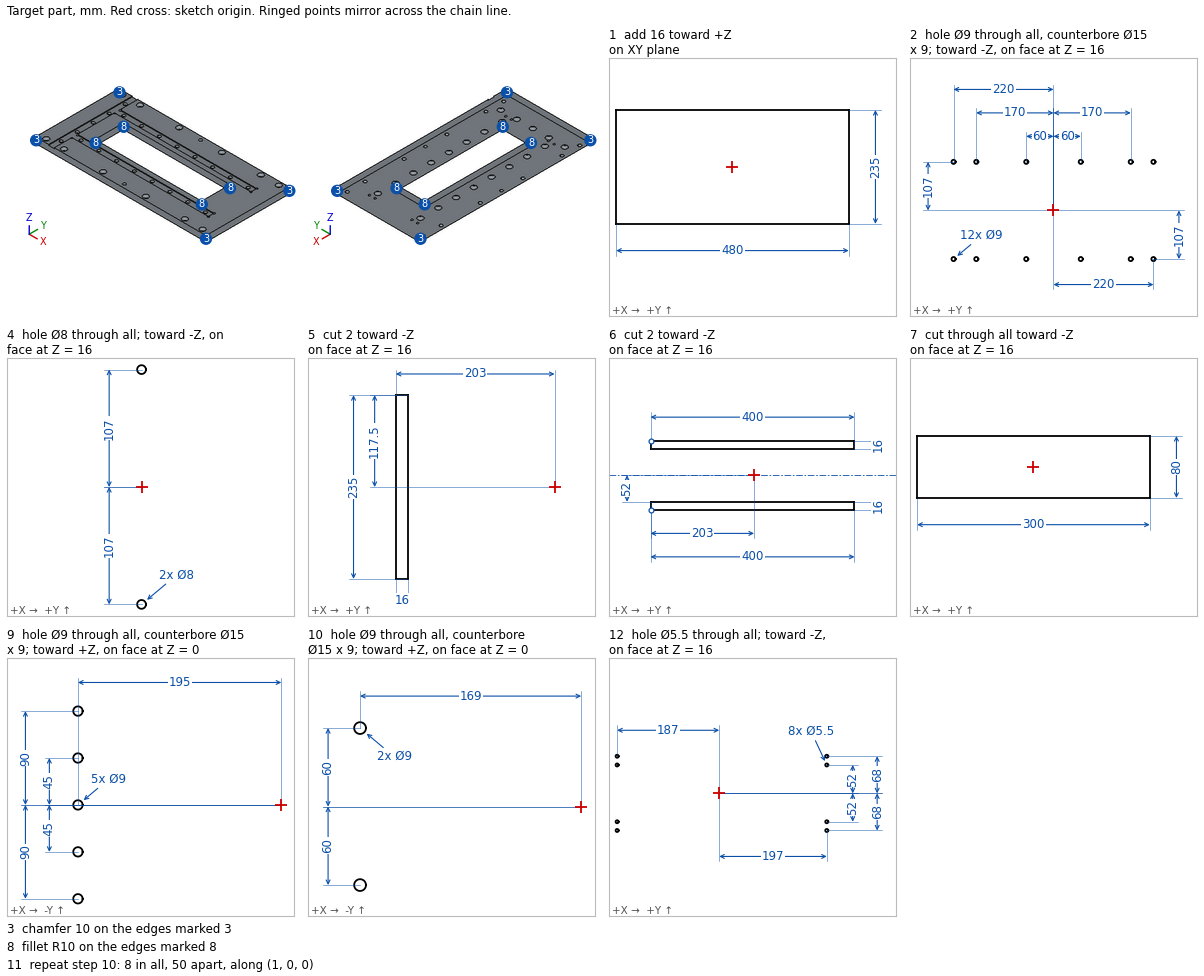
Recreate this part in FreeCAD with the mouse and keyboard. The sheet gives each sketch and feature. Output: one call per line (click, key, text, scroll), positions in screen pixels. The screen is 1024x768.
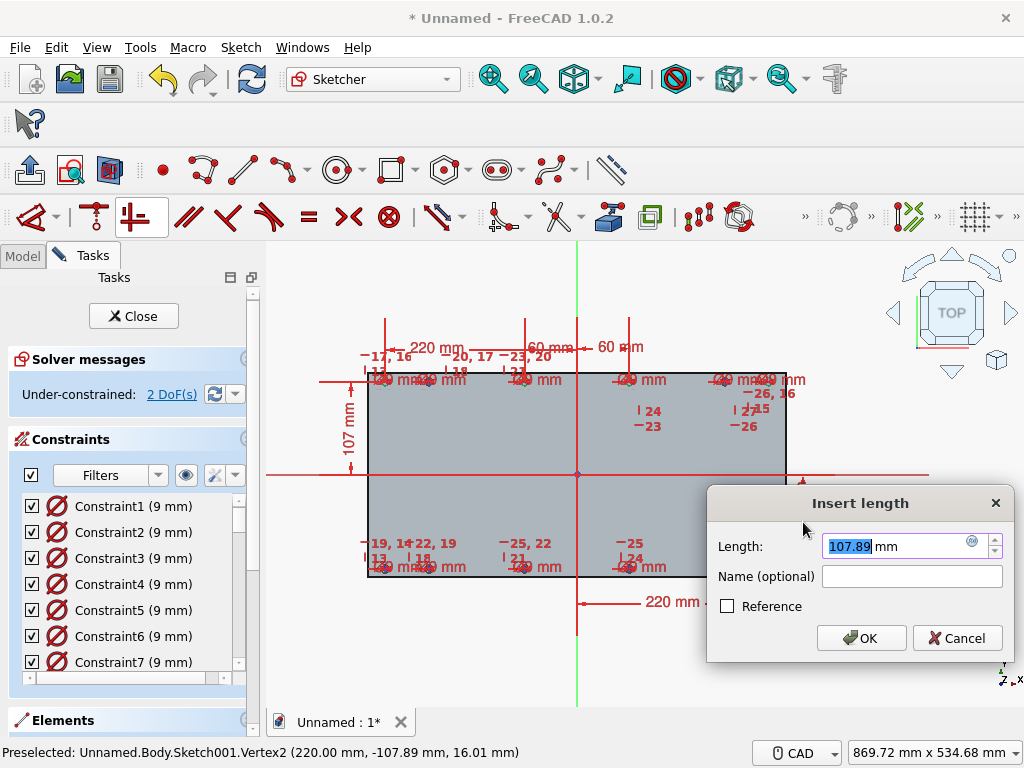
text(107)
key(Return)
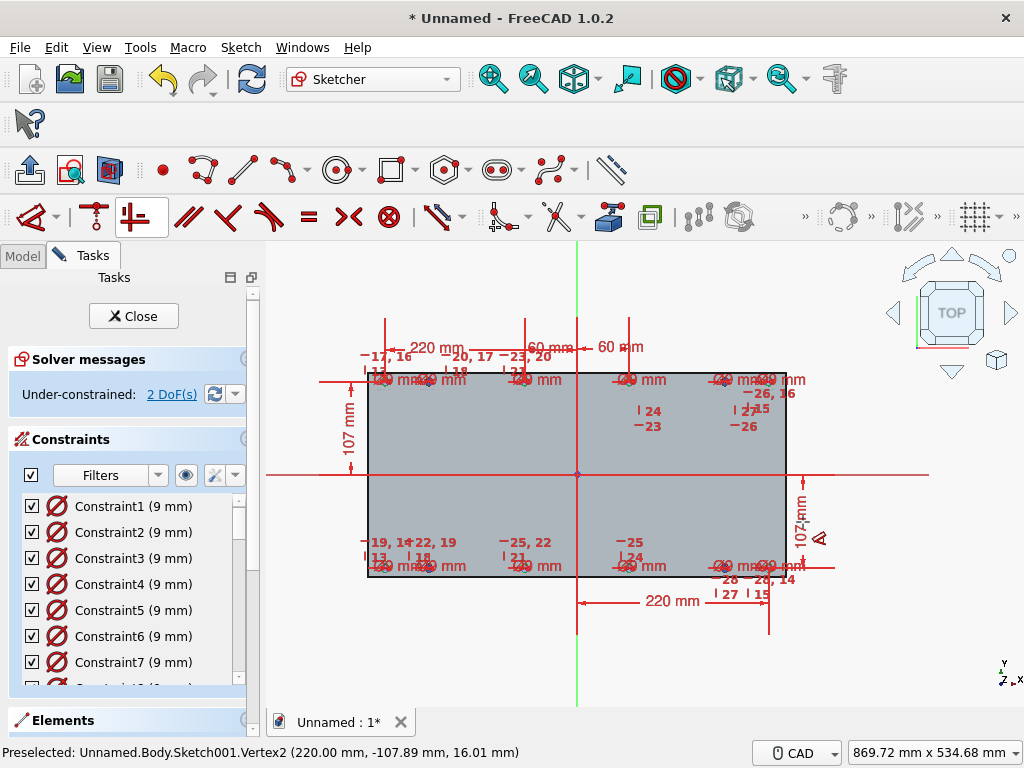
click(429, 382)
click(503, 509)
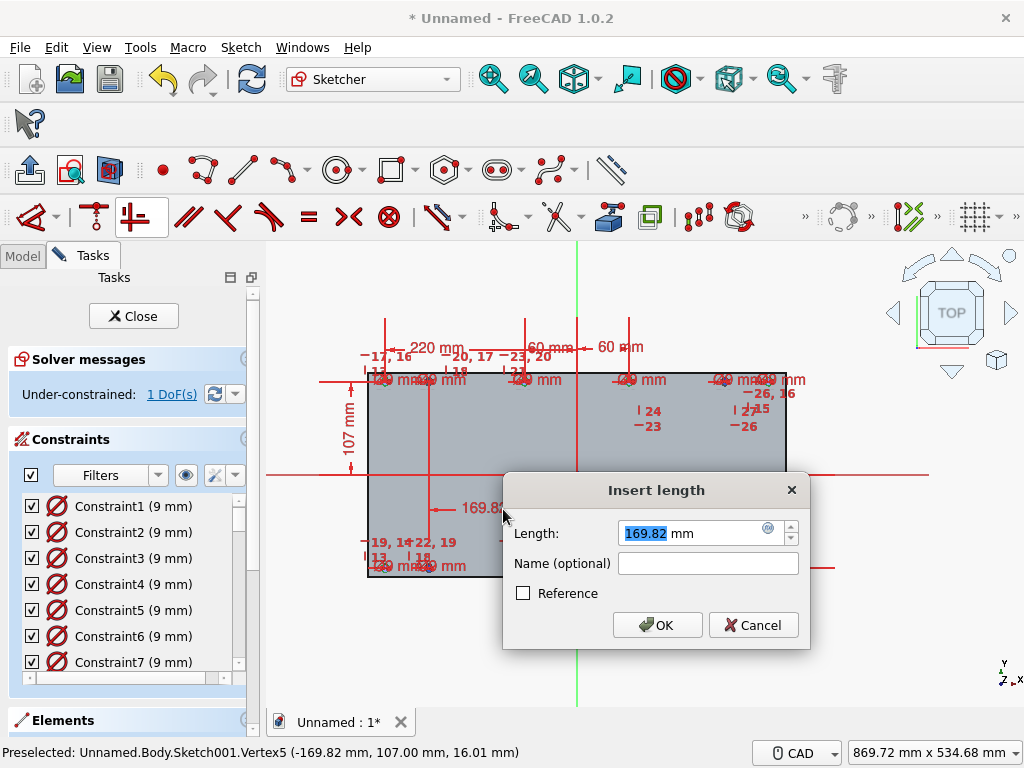
text(170)
key(Return)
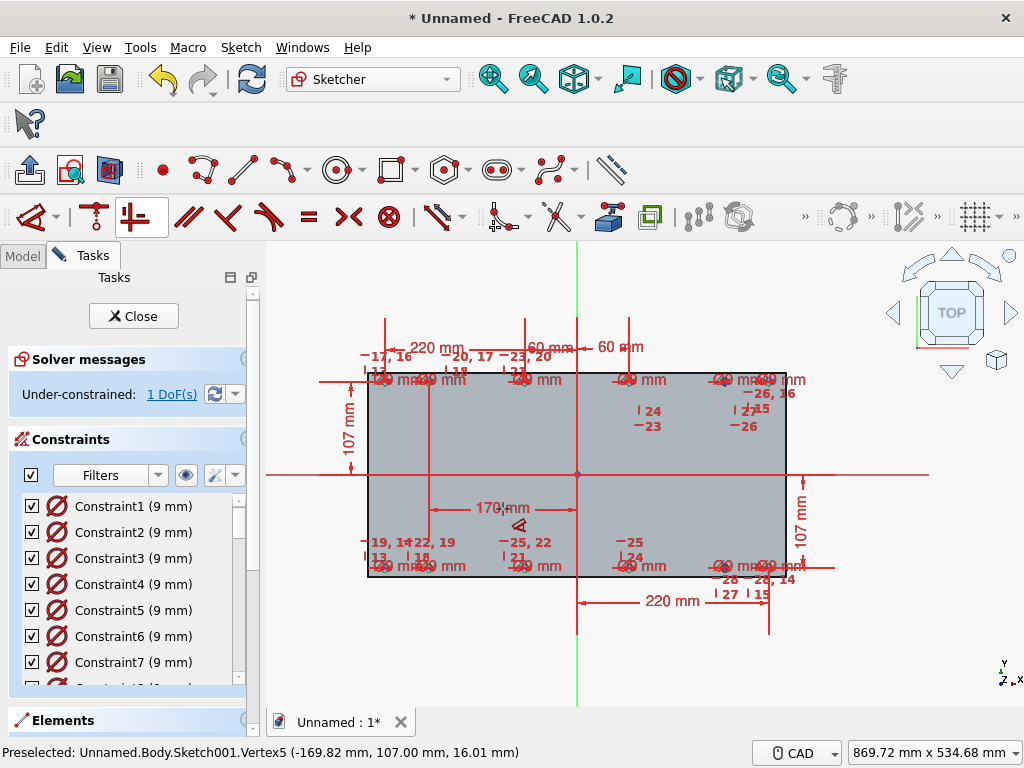
click(725, 382)
click(703, 348)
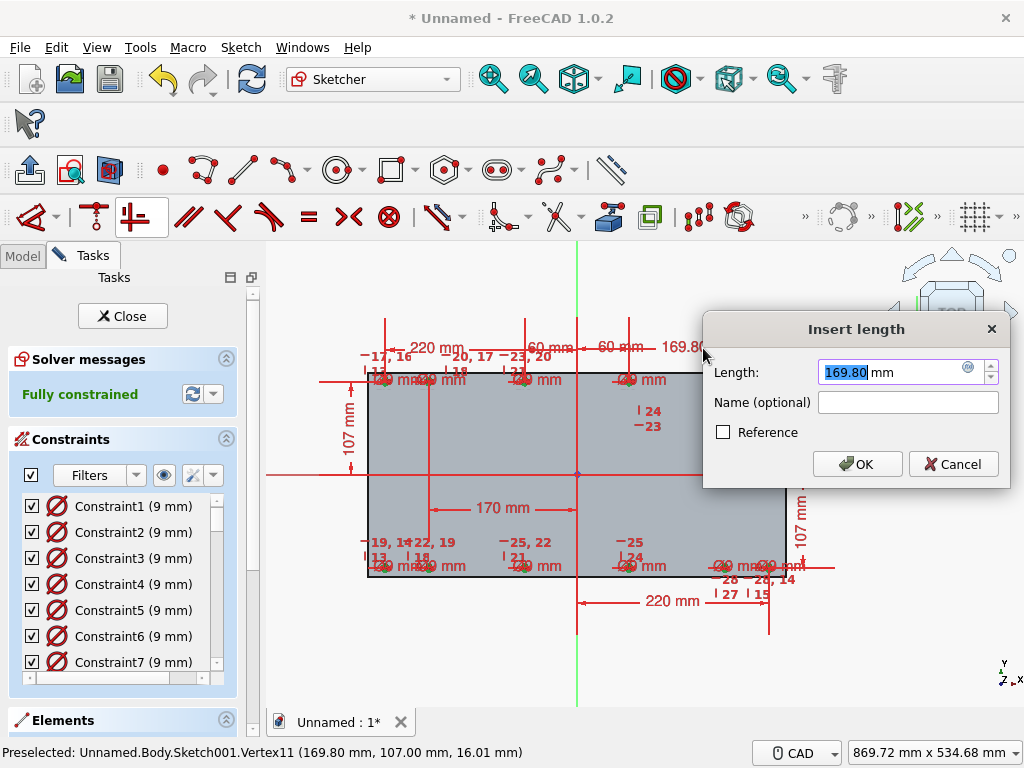
text(170)
key(Return)
key(Escape)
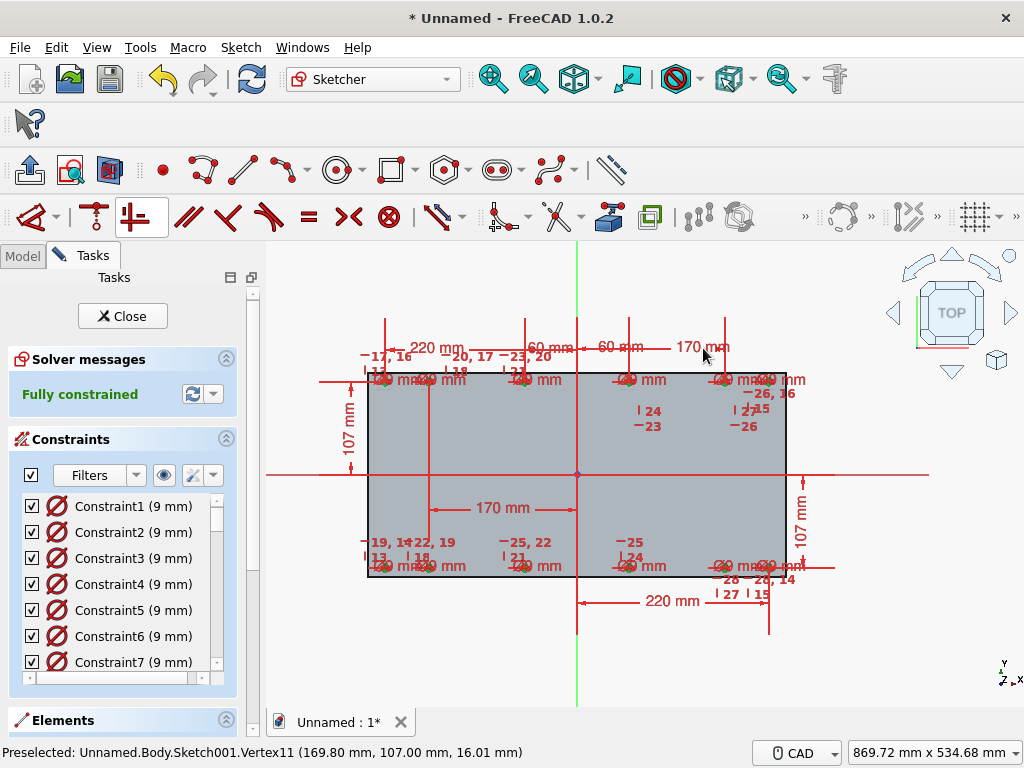
click(123, 316)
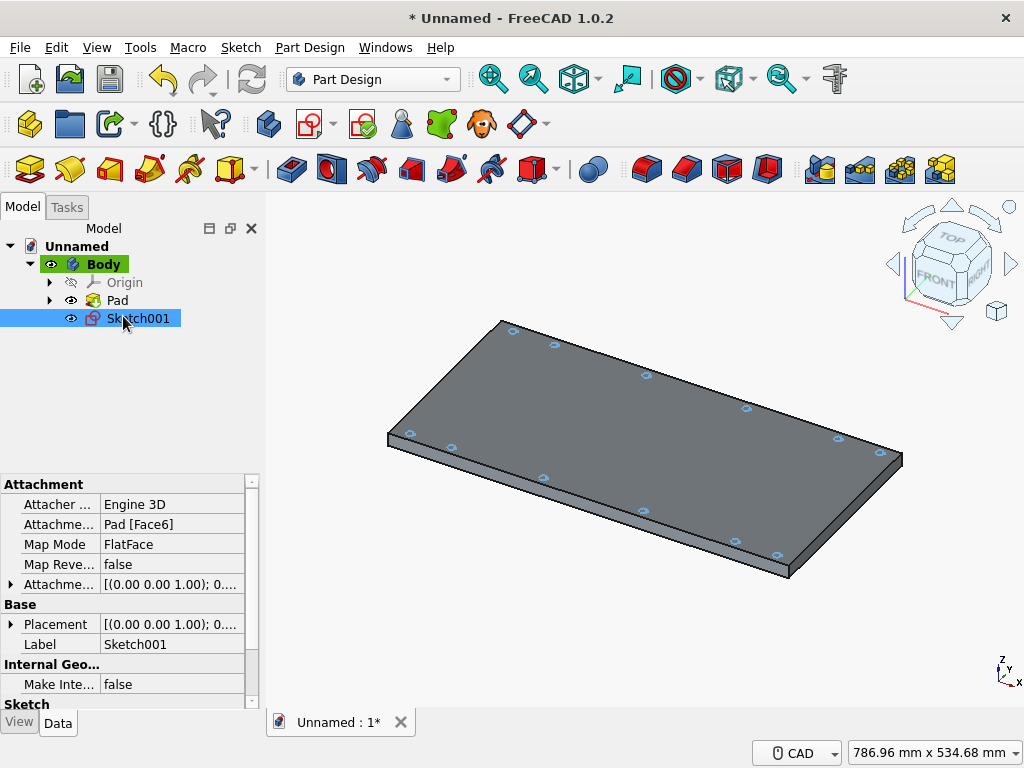
click(332, 170)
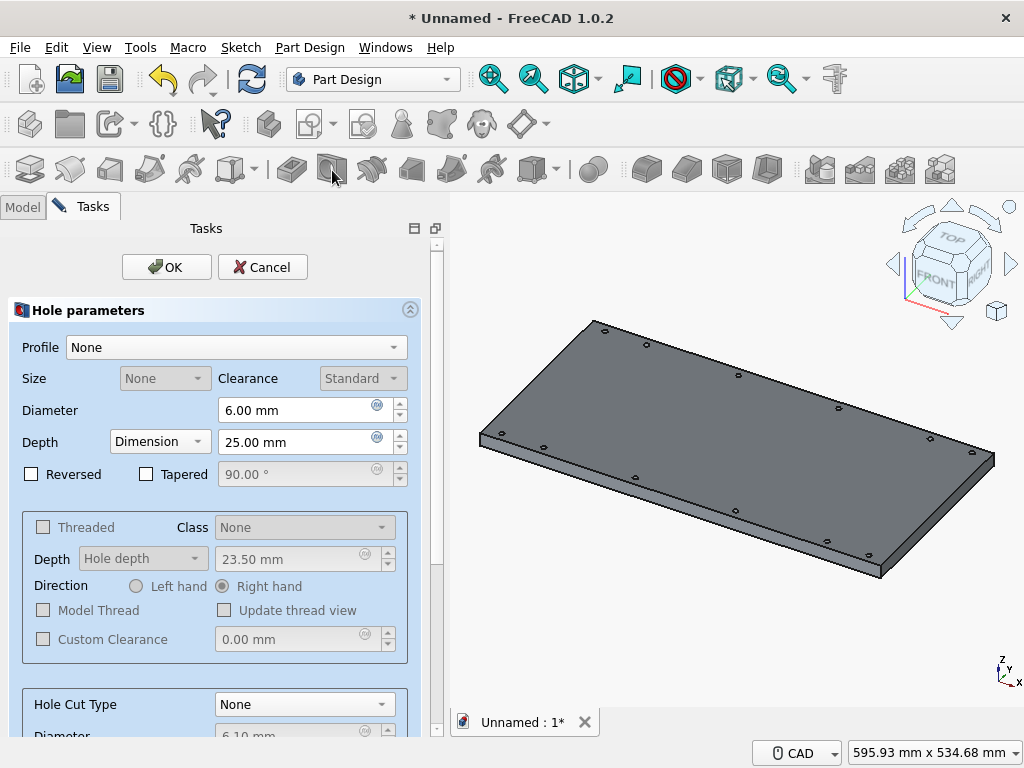
triple_click(305, 410)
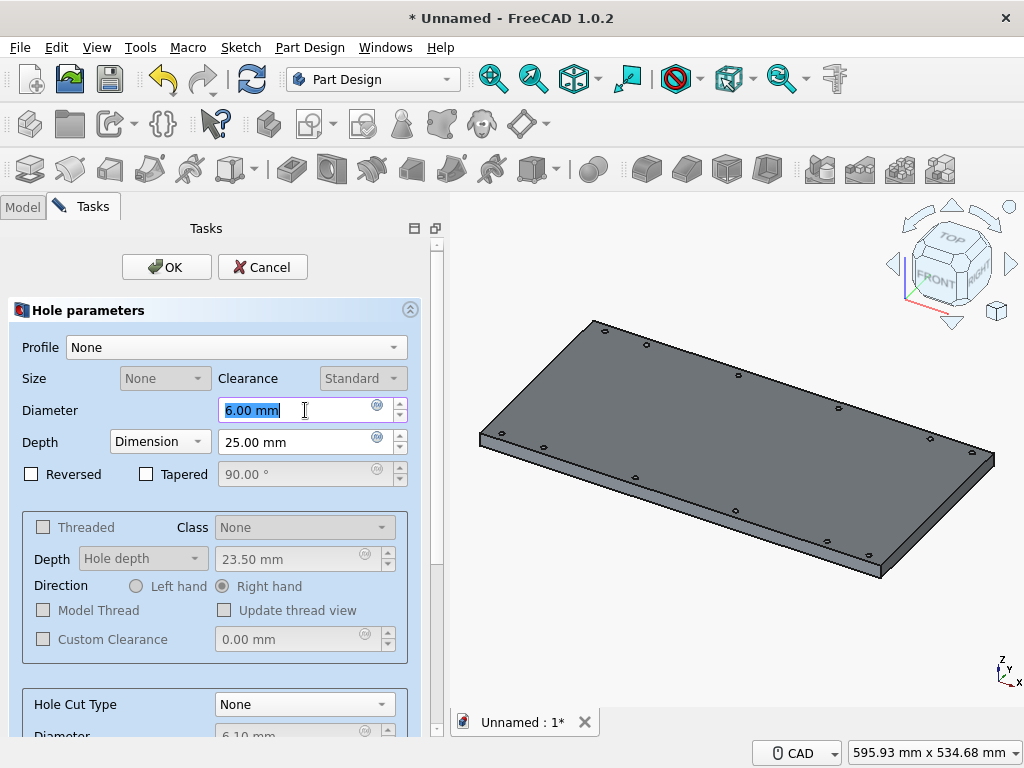
text(9)
key(Tab)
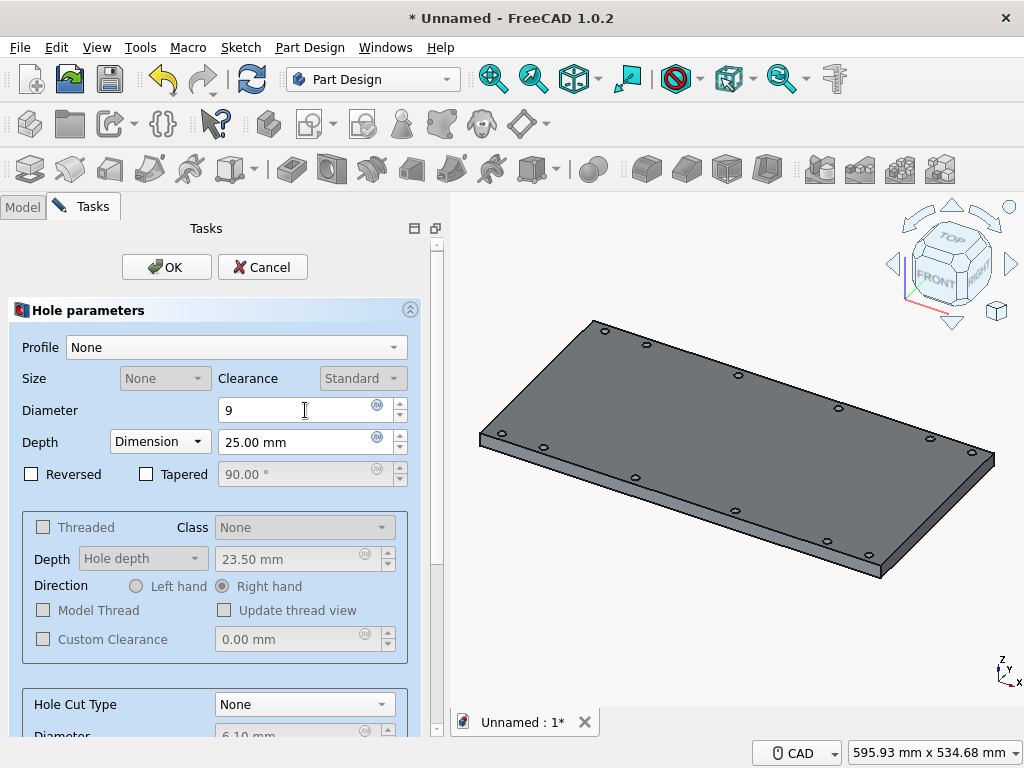
click(161, 442)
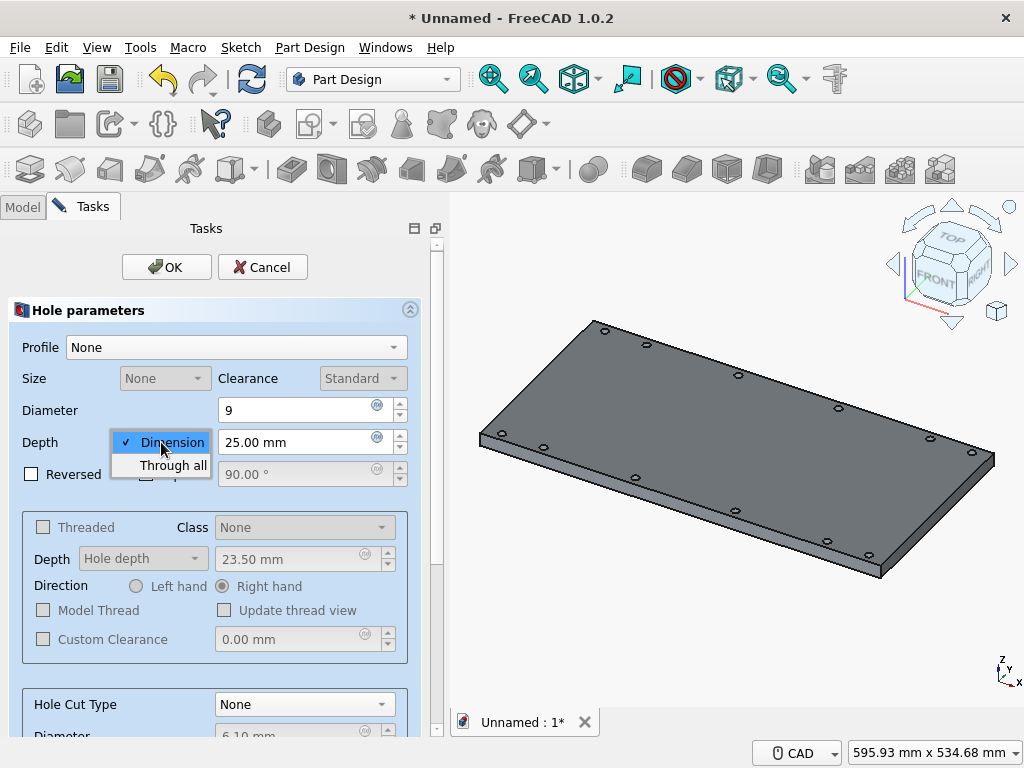
click(160, 466)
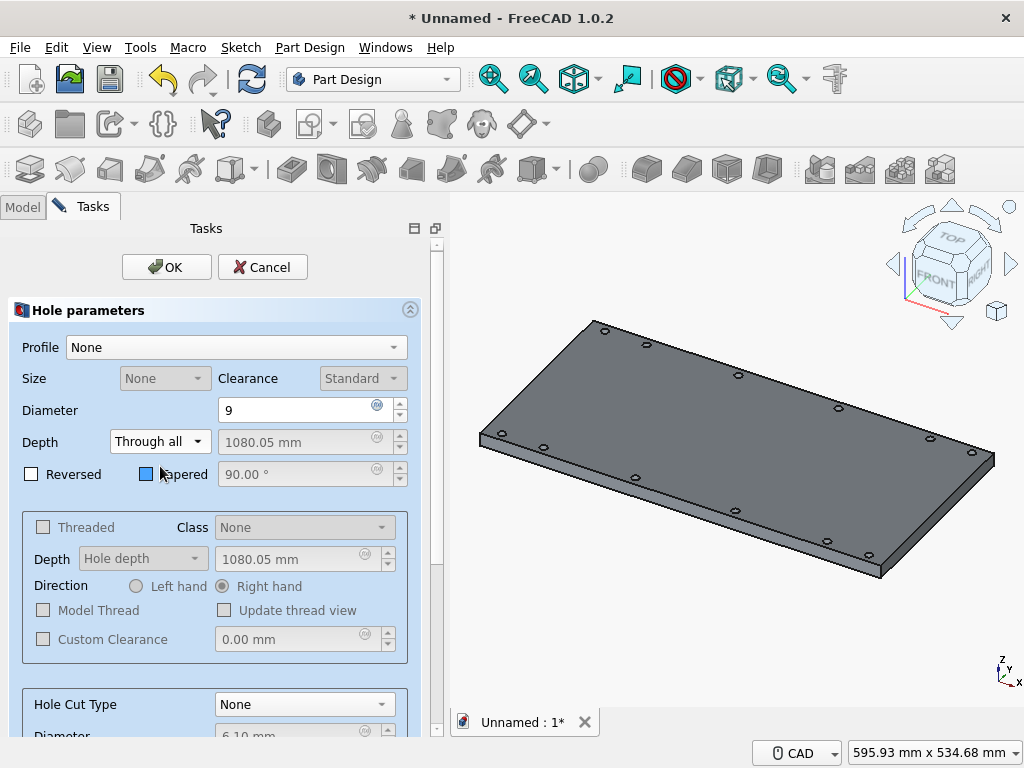
click(306, 704)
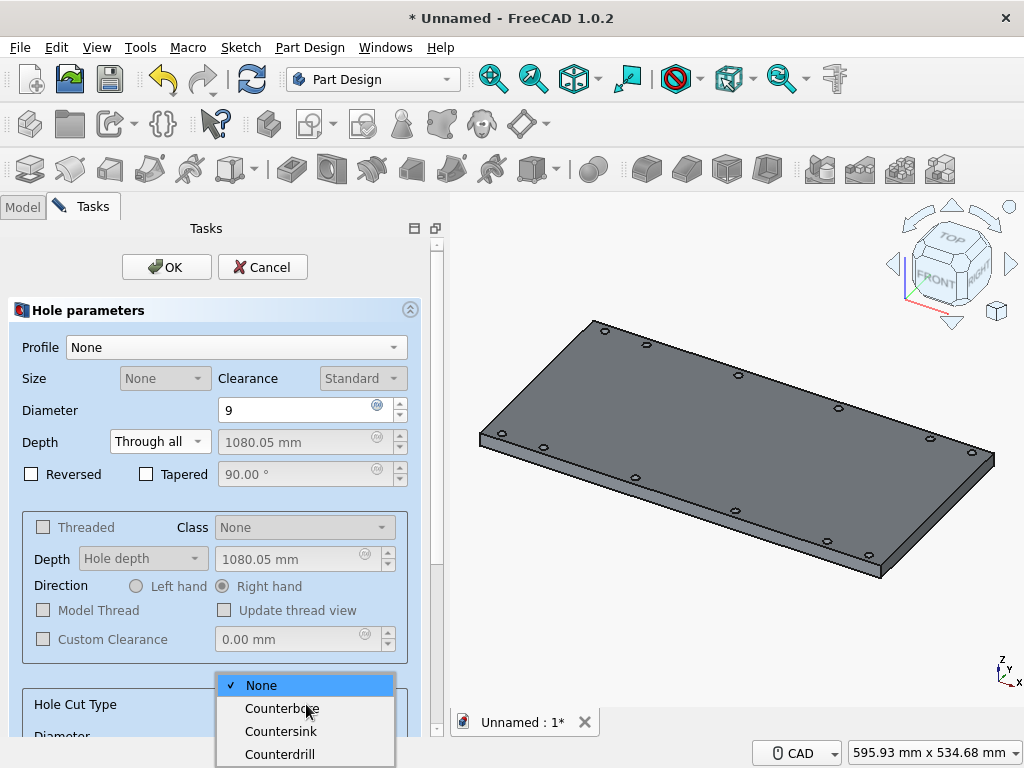
click(304, 708)